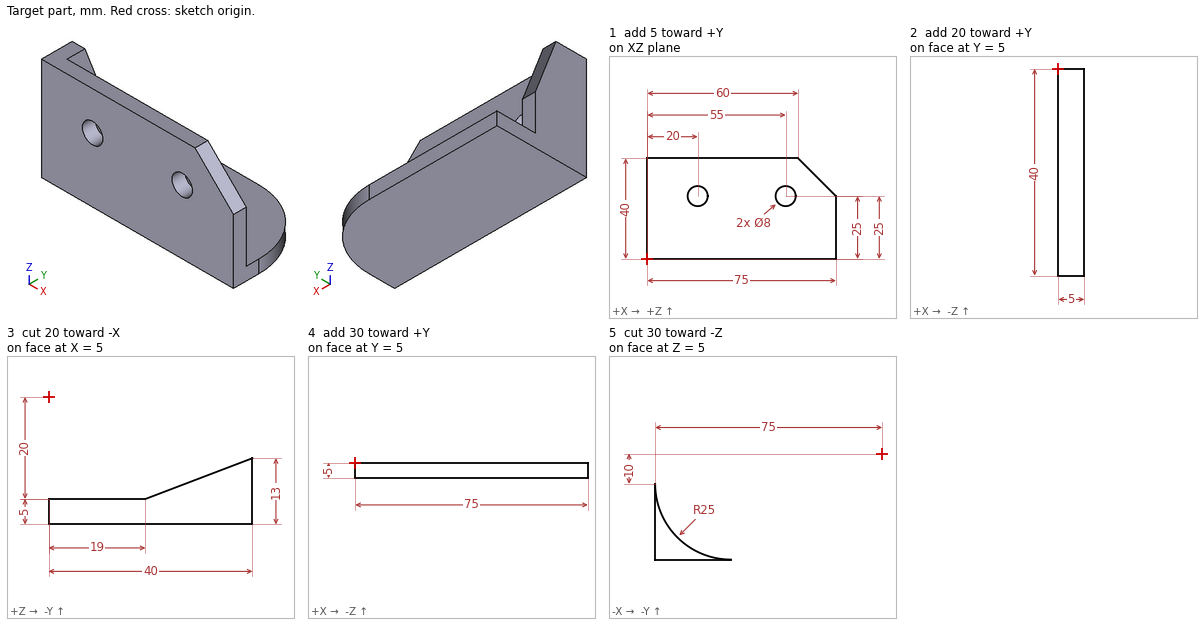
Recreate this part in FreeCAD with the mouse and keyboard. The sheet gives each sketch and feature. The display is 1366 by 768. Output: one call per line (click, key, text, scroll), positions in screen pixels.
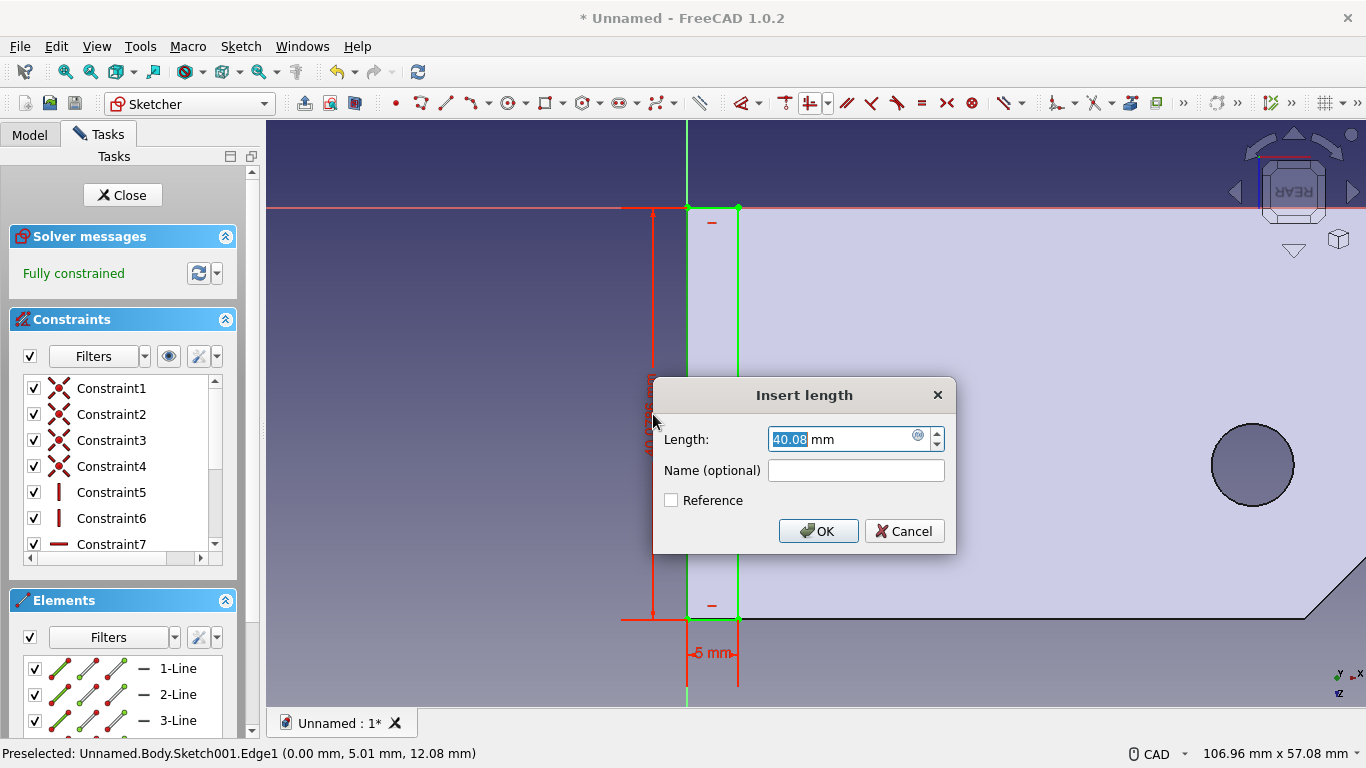
text(40)
key(Return)
key(Escape)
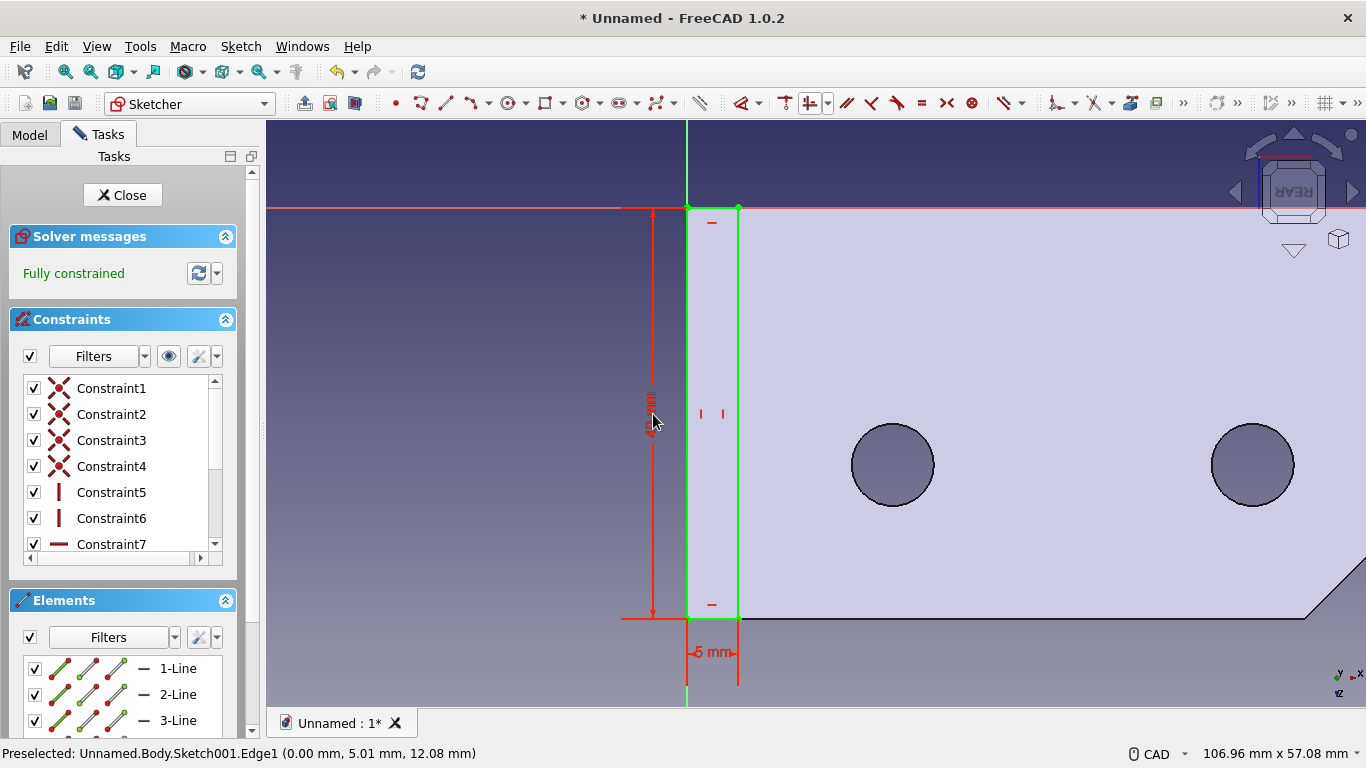
click(123, 195)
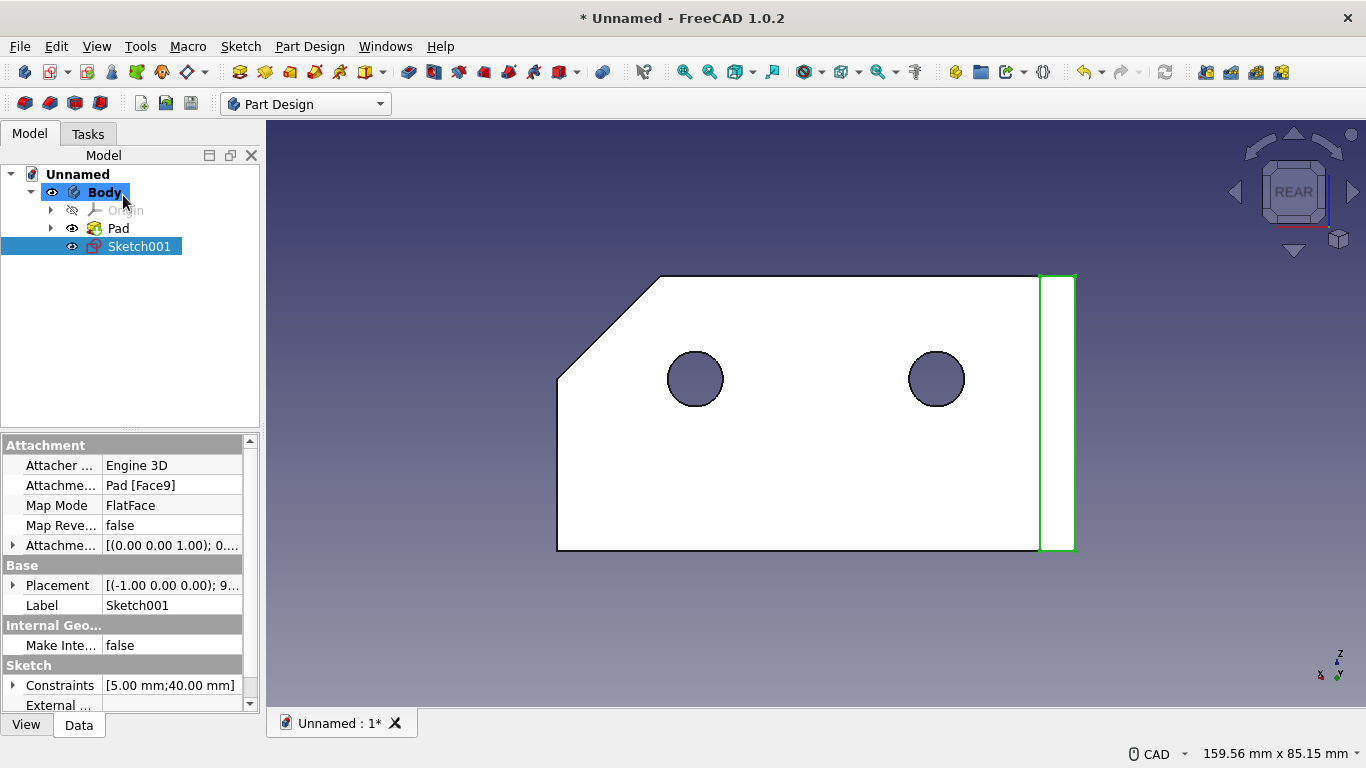
click(240, 72)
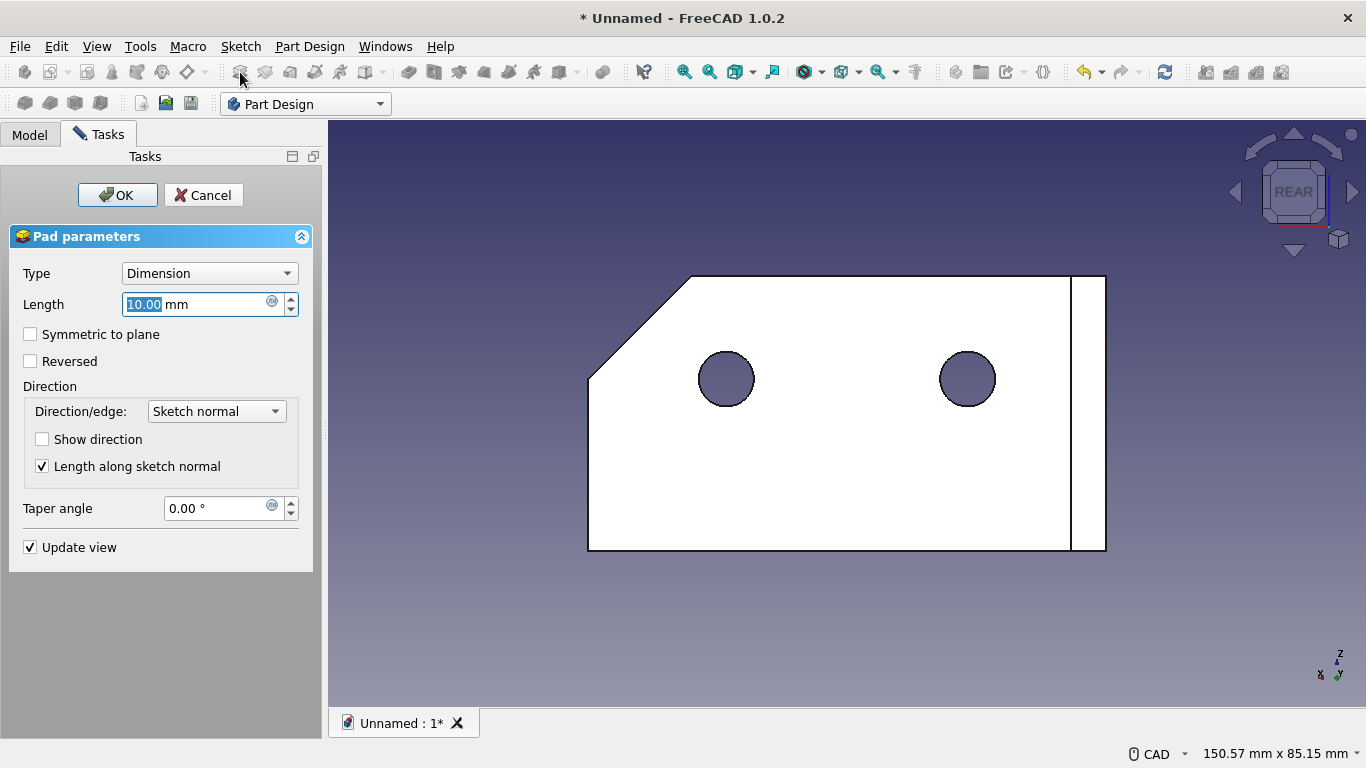
text(20)
key(Tab)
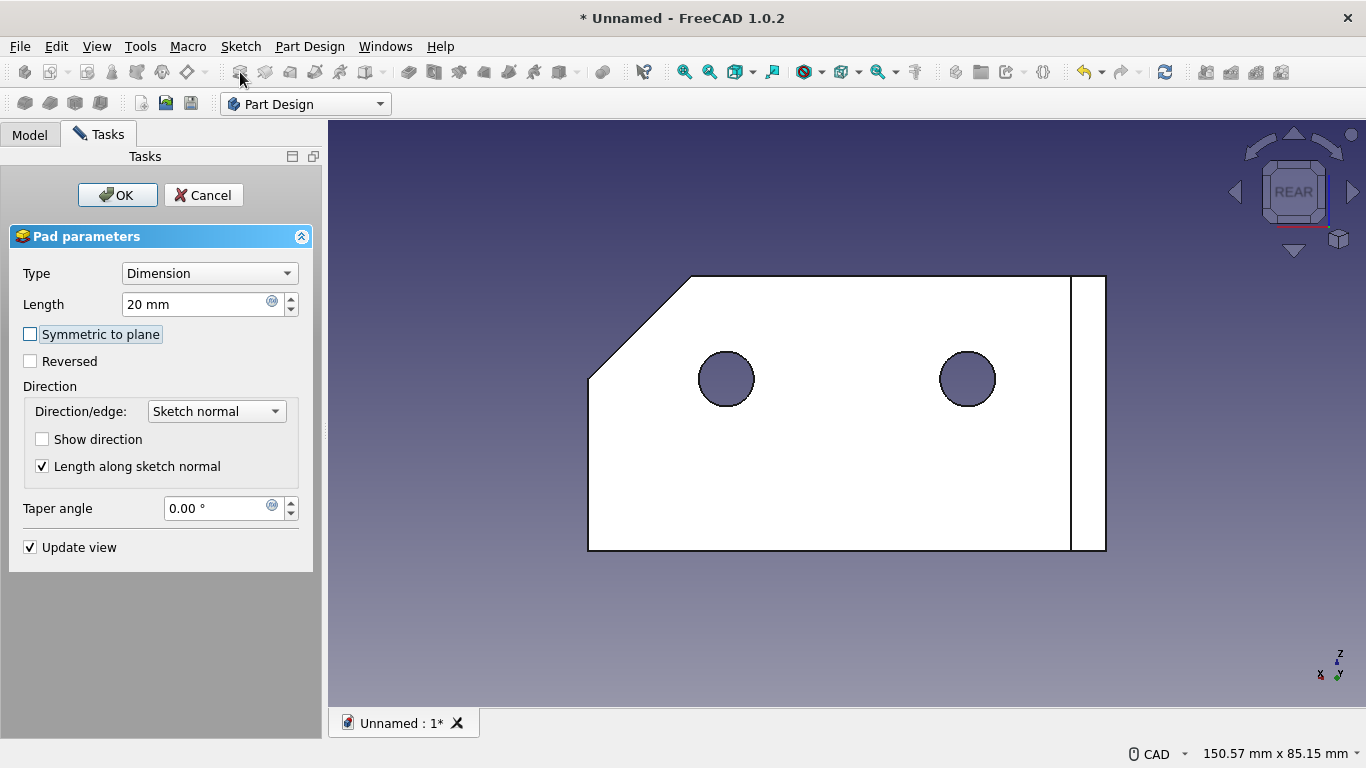
click(118, 195)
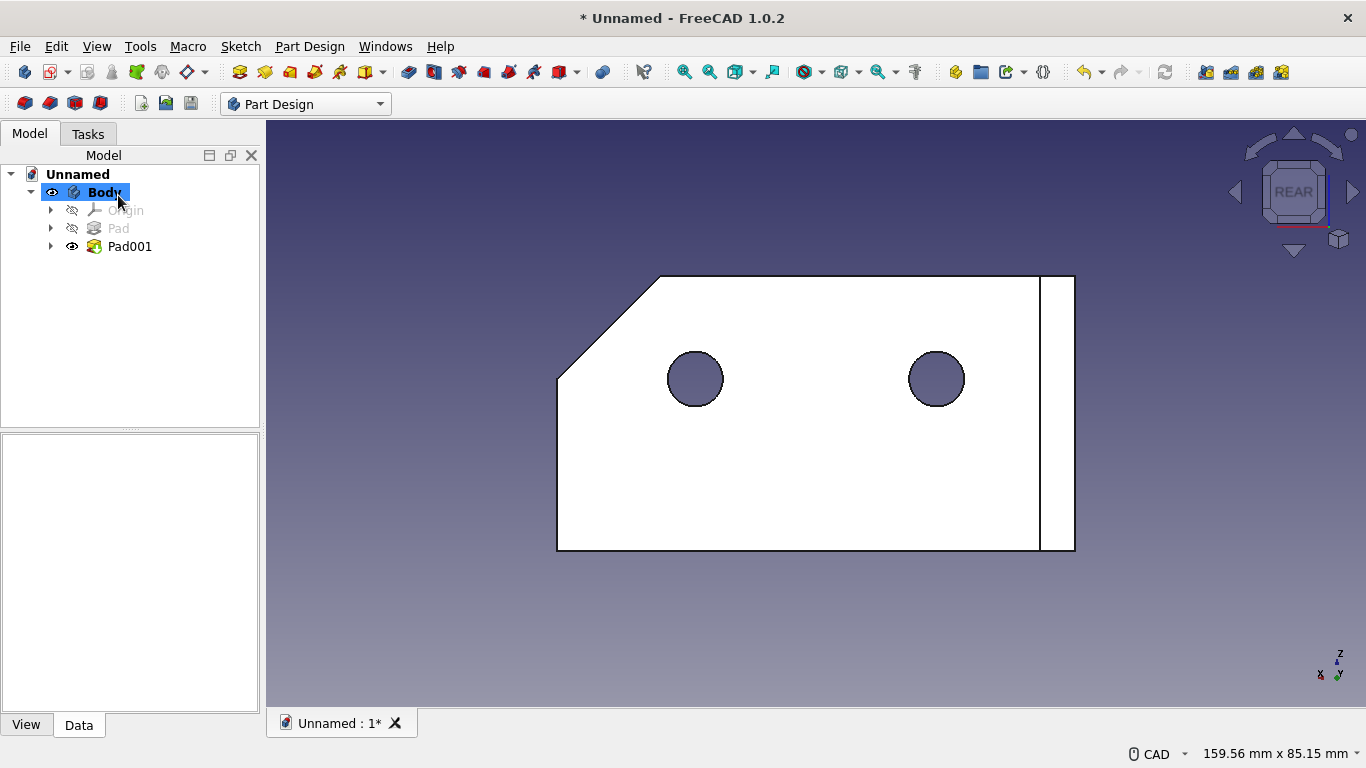
key(0)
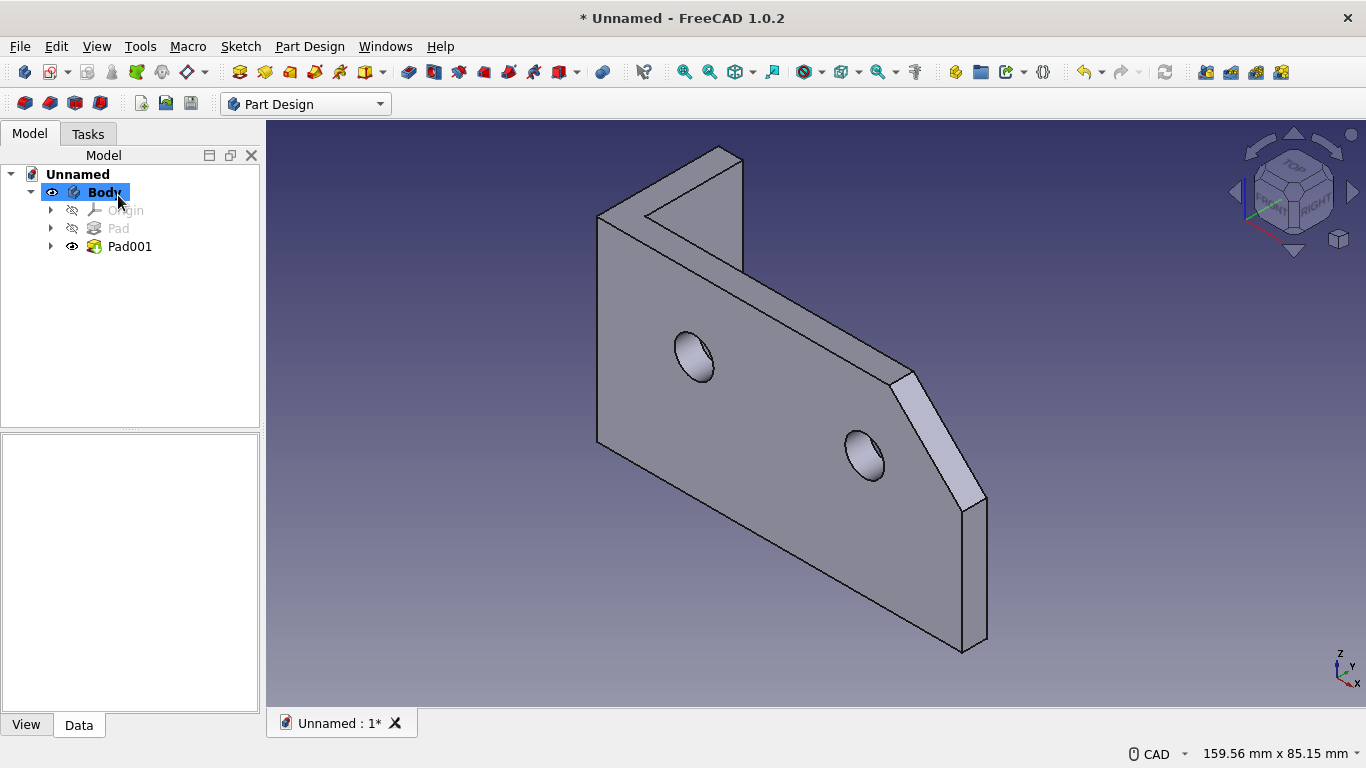
click(708, 228)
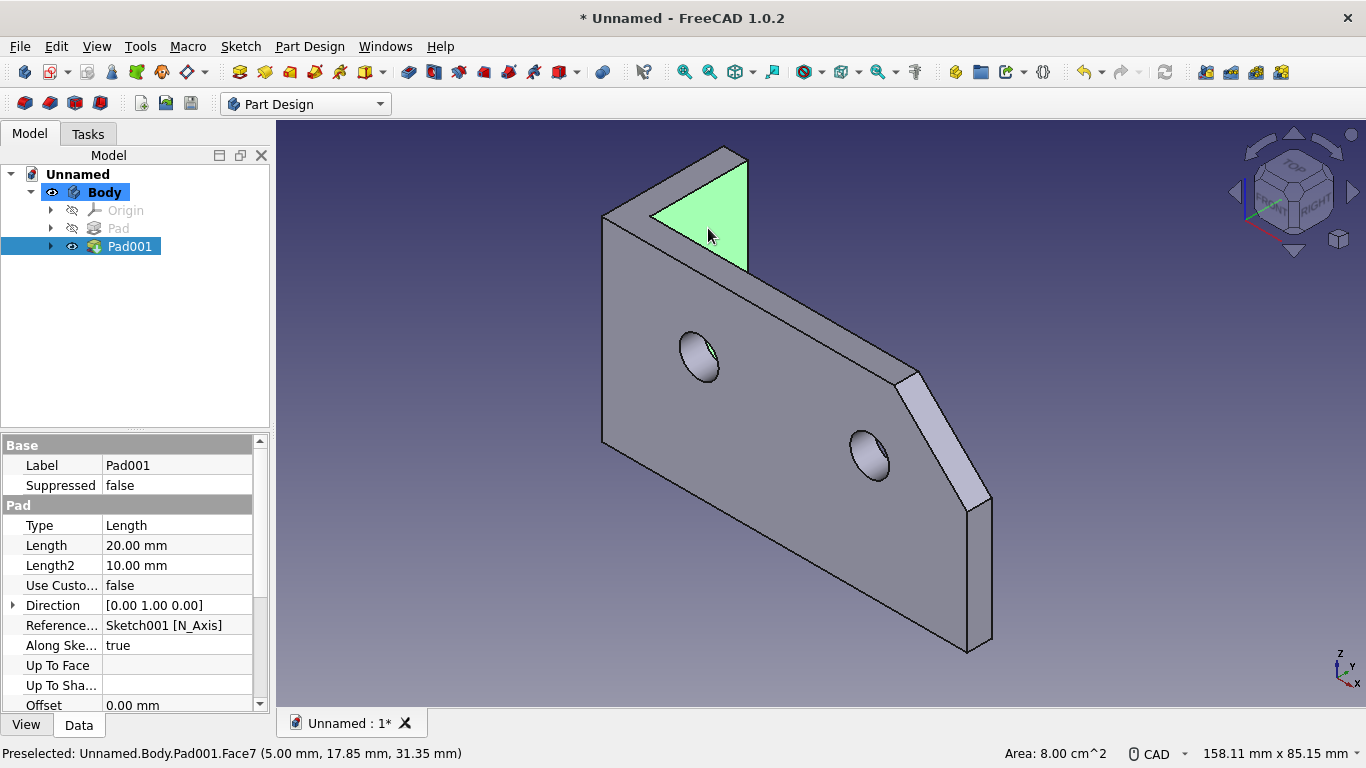
click(50, 72)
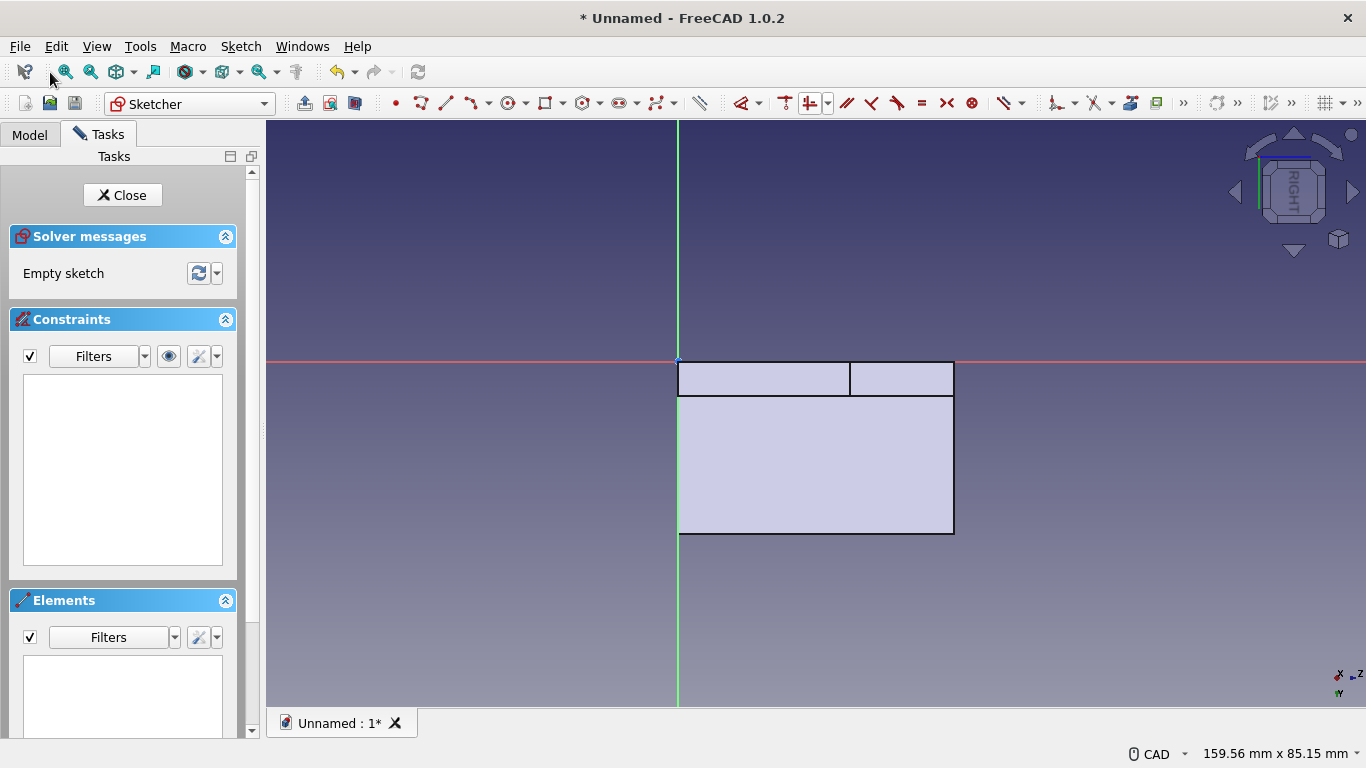
scroll(872, 476, up, 4)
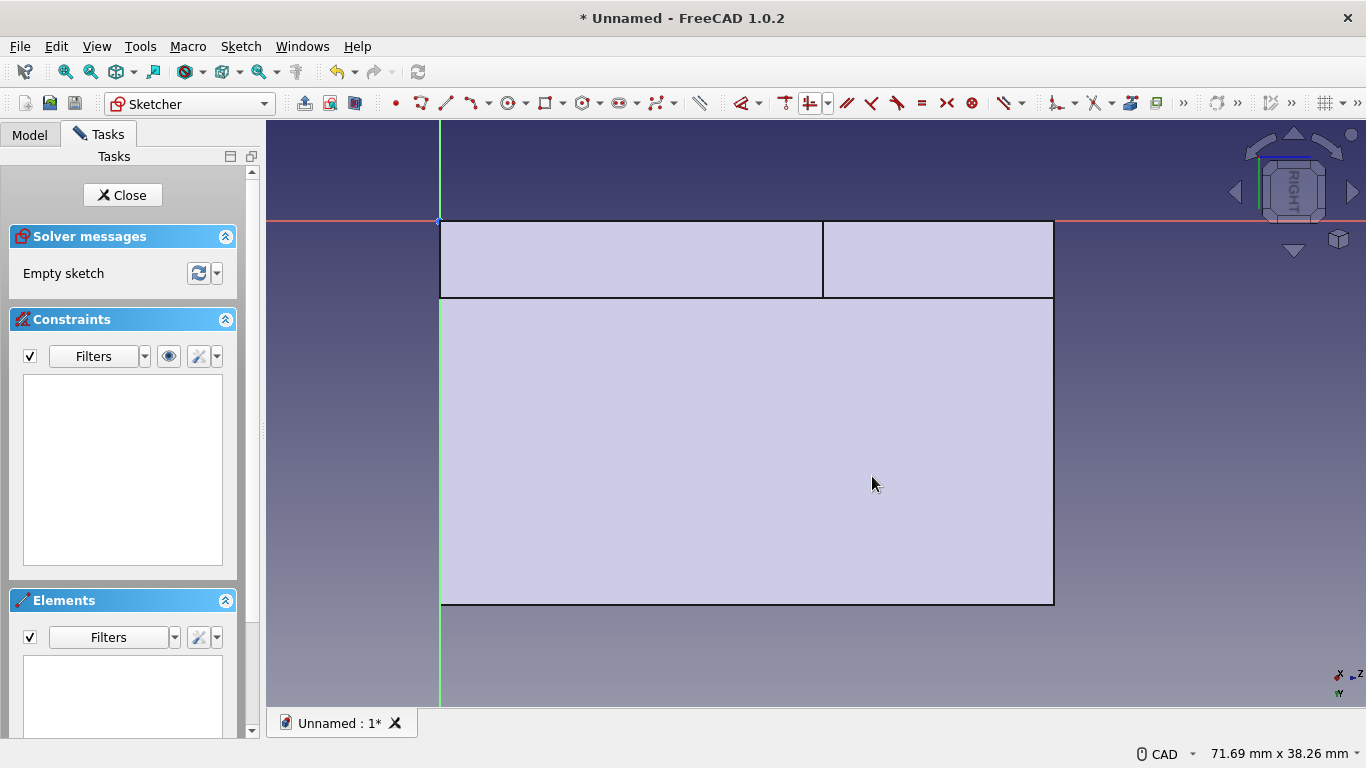
click(421, 104)